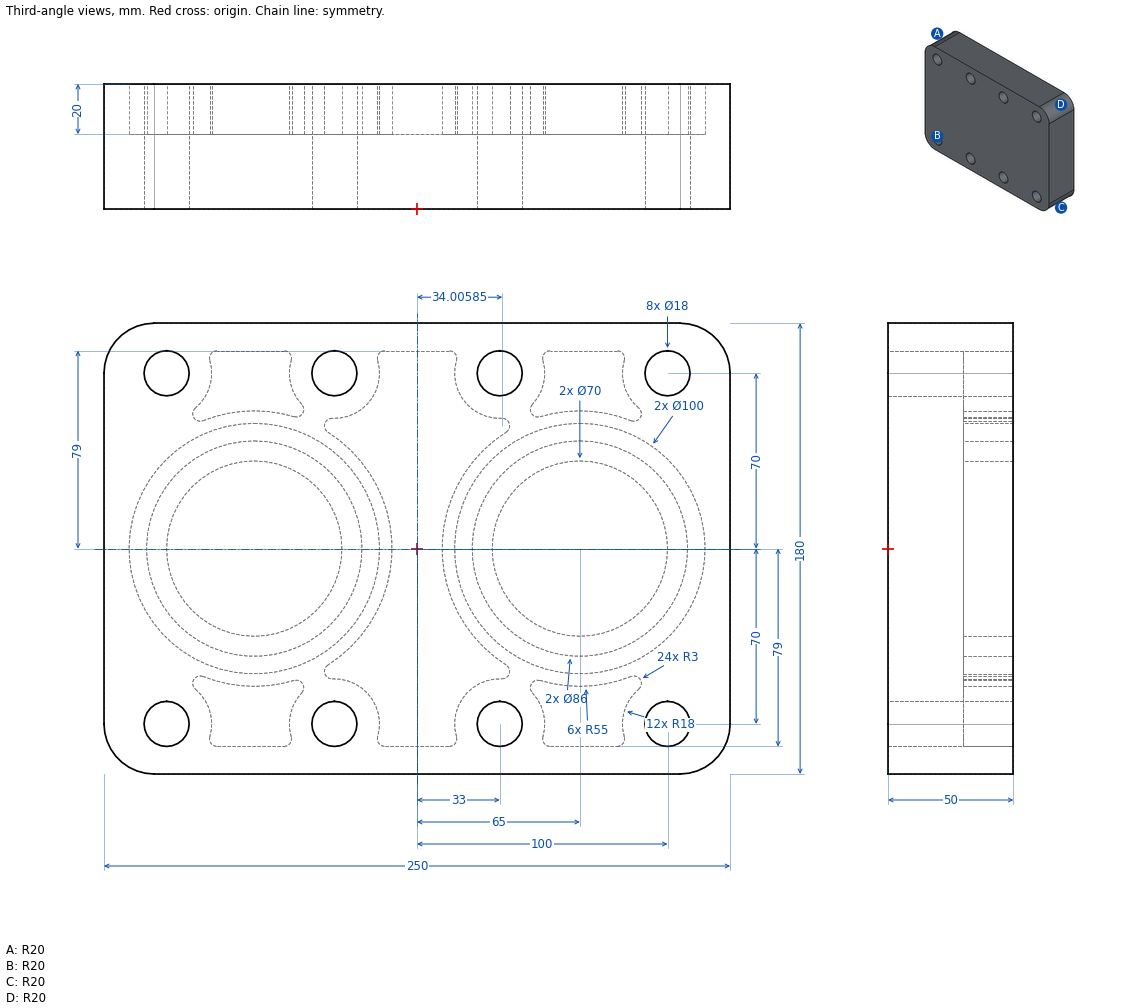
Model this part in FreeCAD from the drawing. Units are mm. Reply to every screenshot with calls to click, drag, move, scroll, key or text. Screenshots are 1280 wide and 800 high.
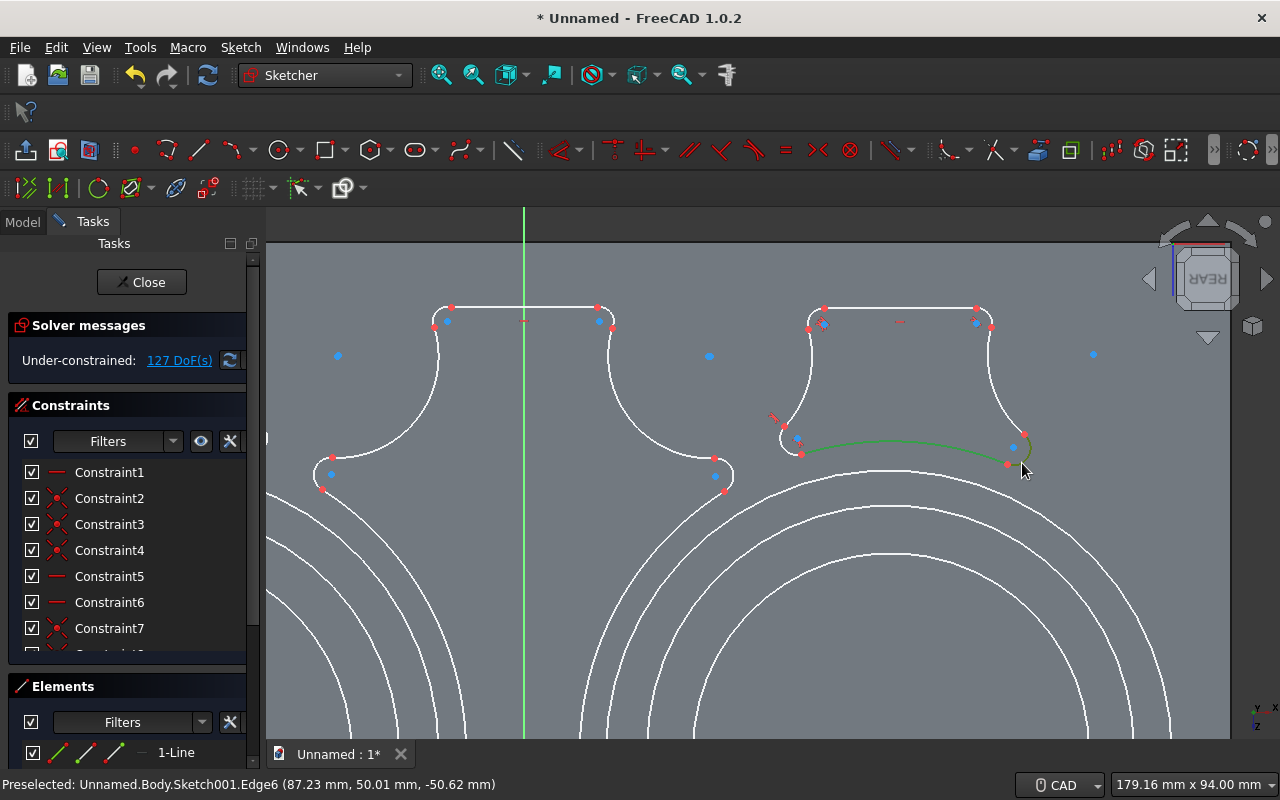
click(754, 150)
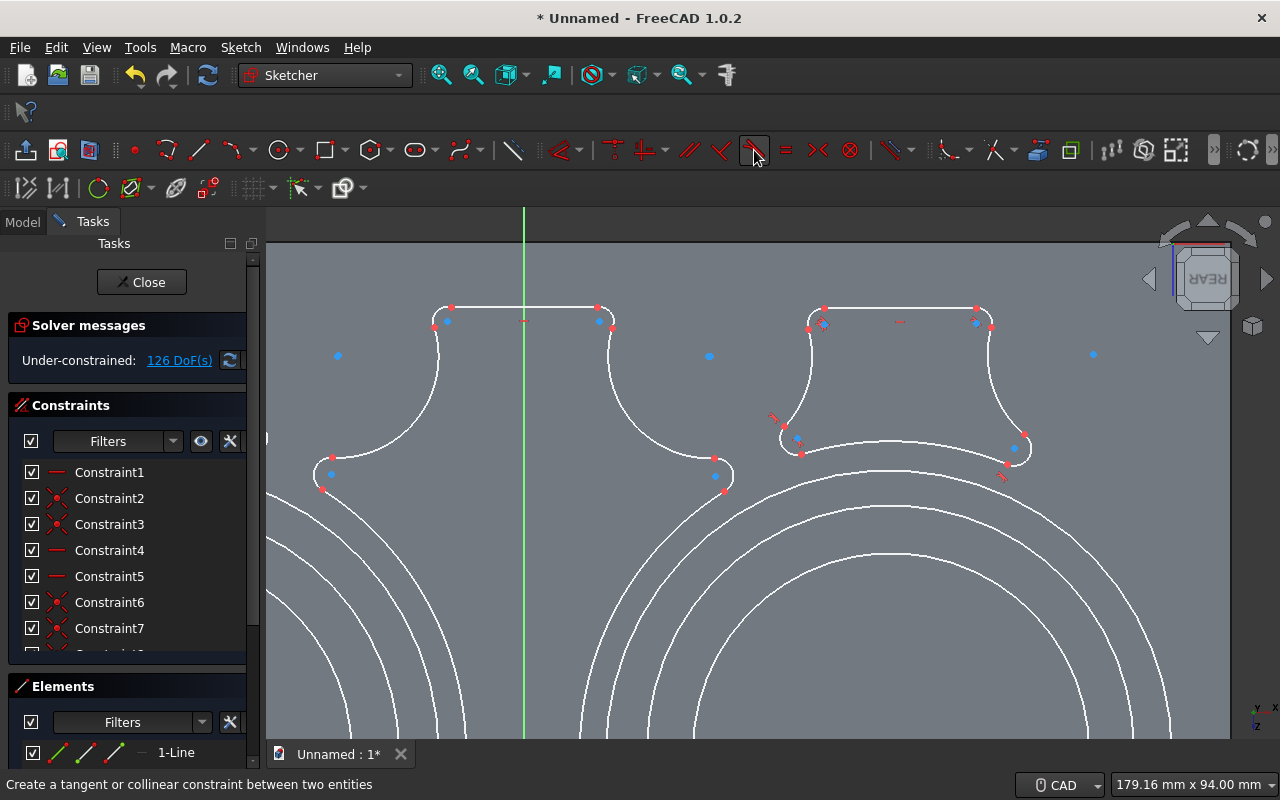
click(1022, 464)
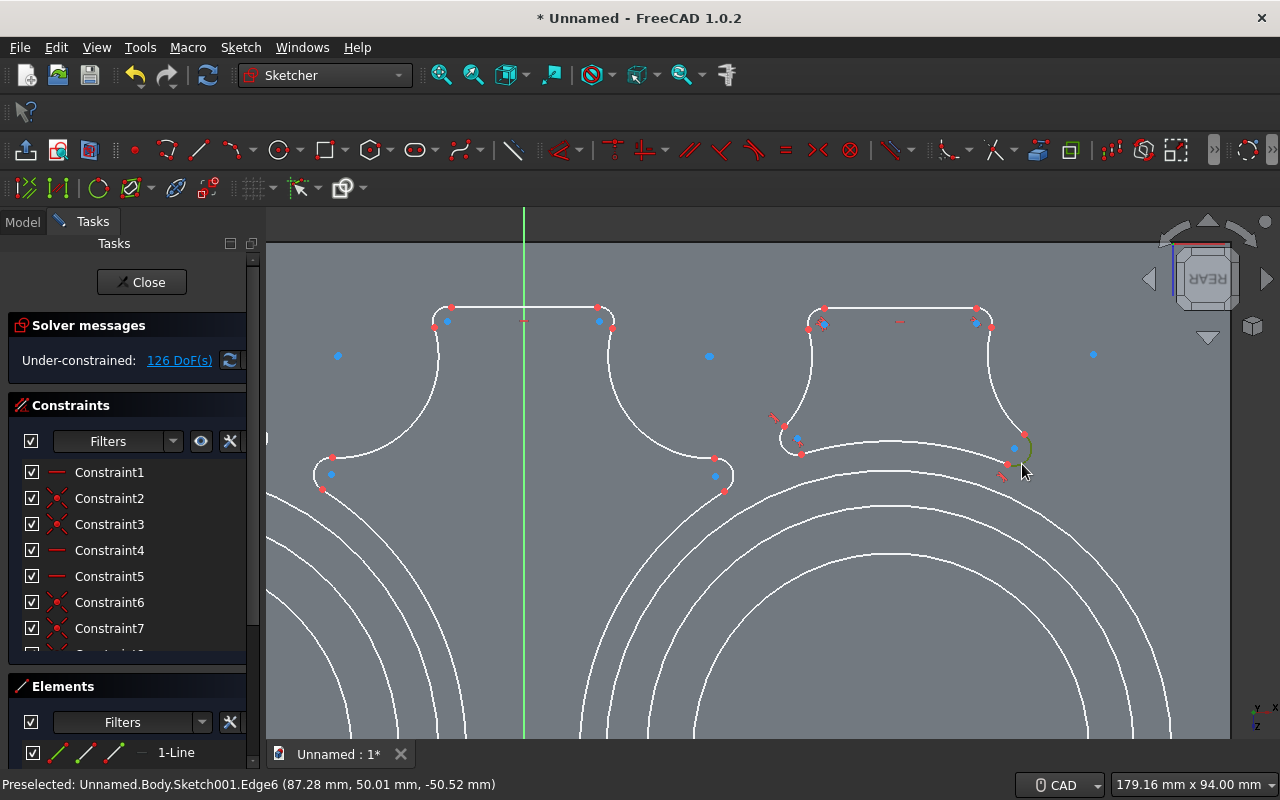
click(988, 362)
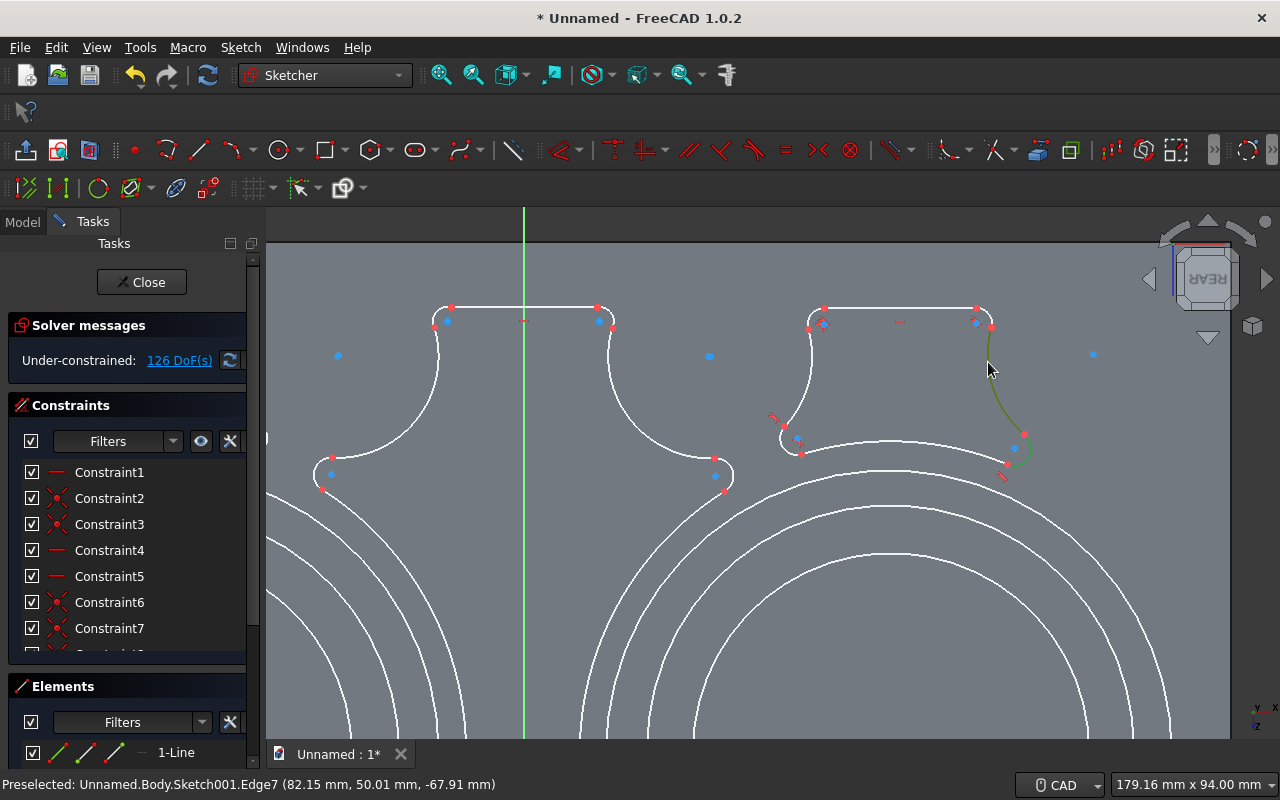
click(754, 150)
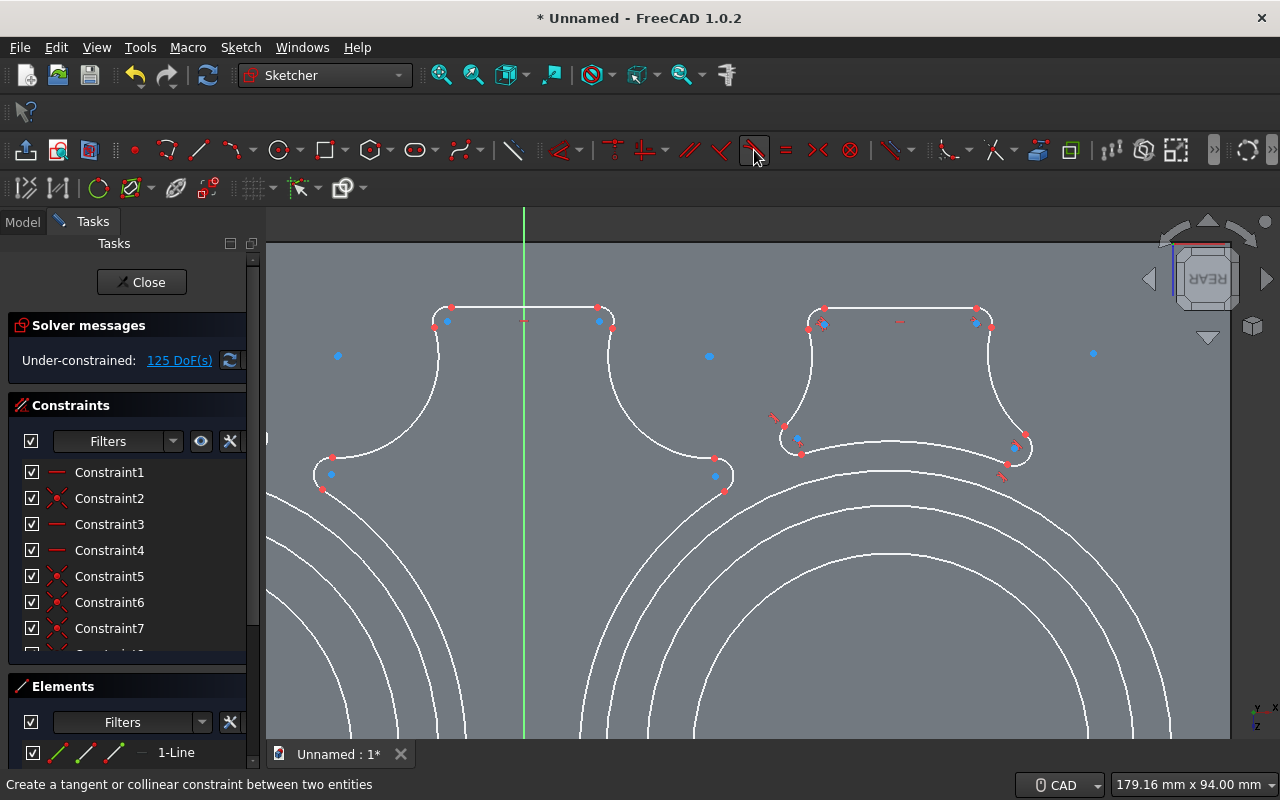
click(988, 362)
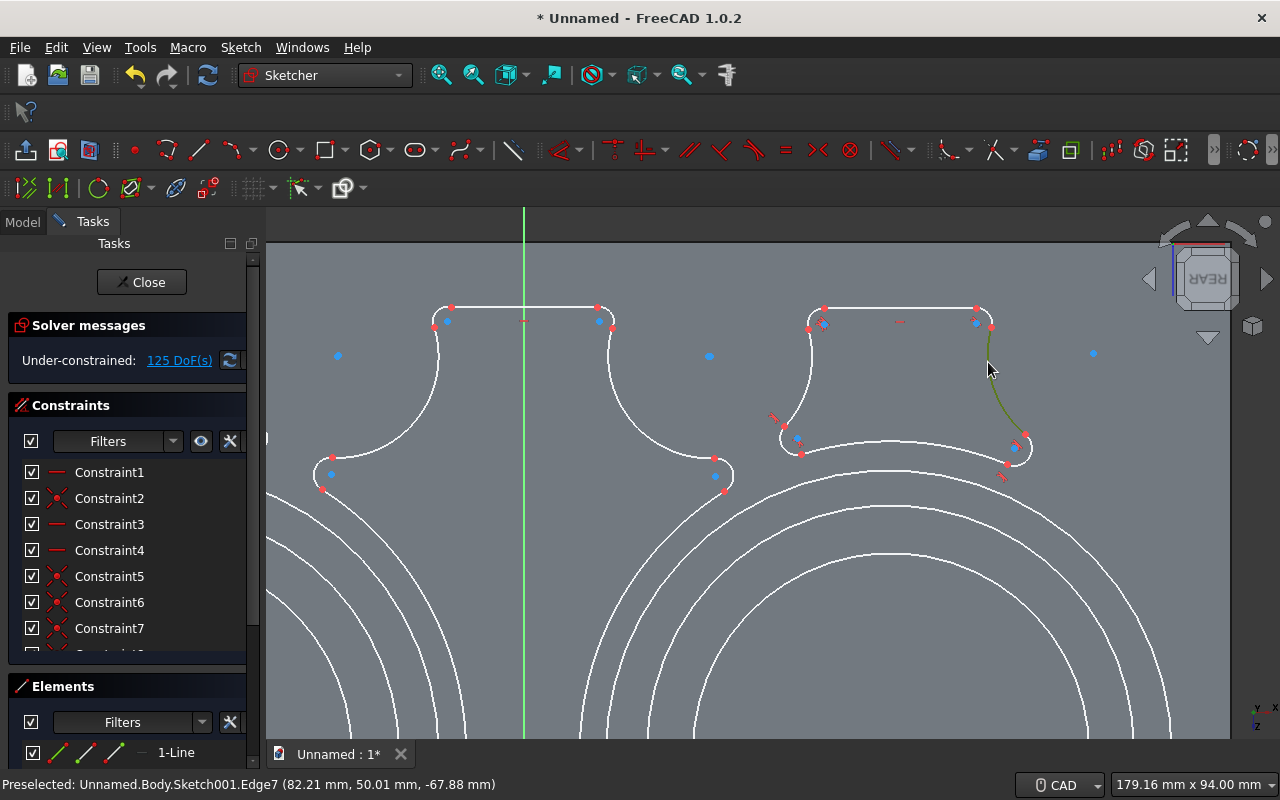
click(989, 314)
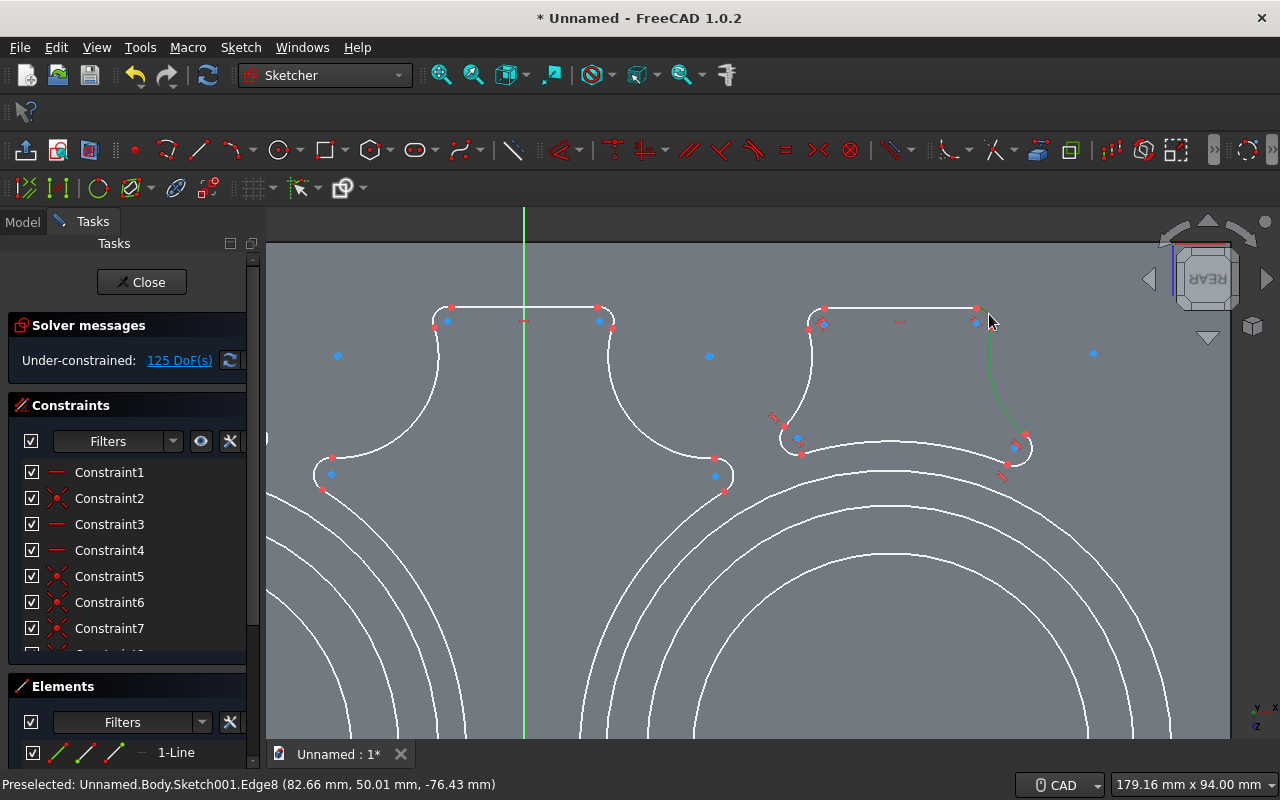
click(754, 150)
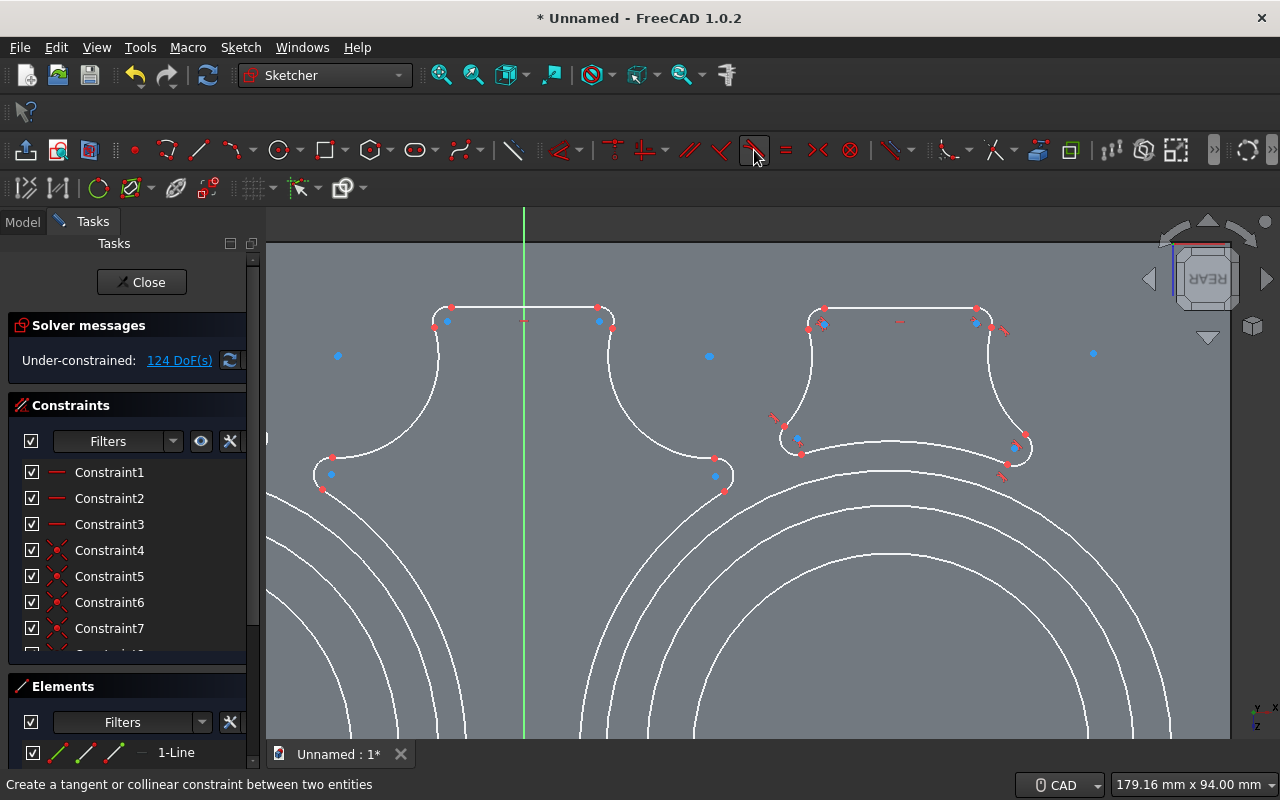
scroll(810, 311, down, 5)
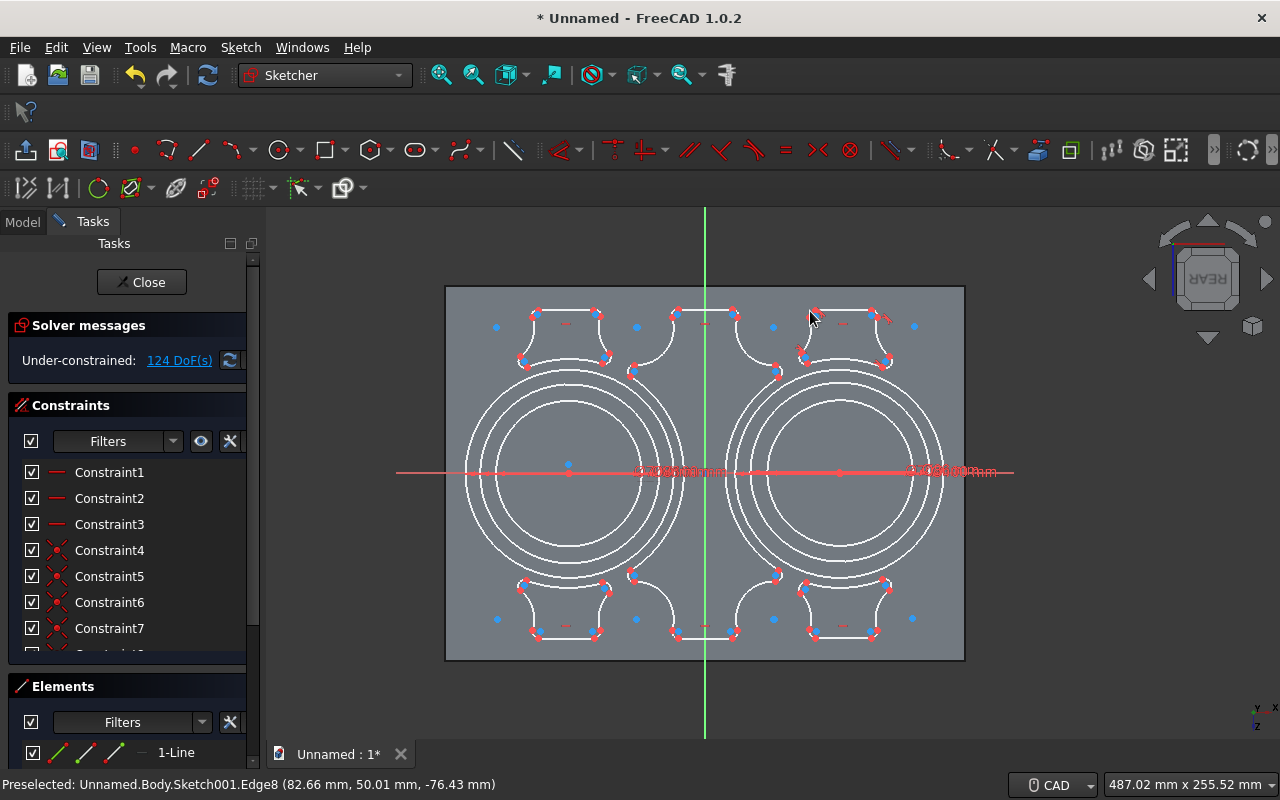
scroll(694, 639, up, 2)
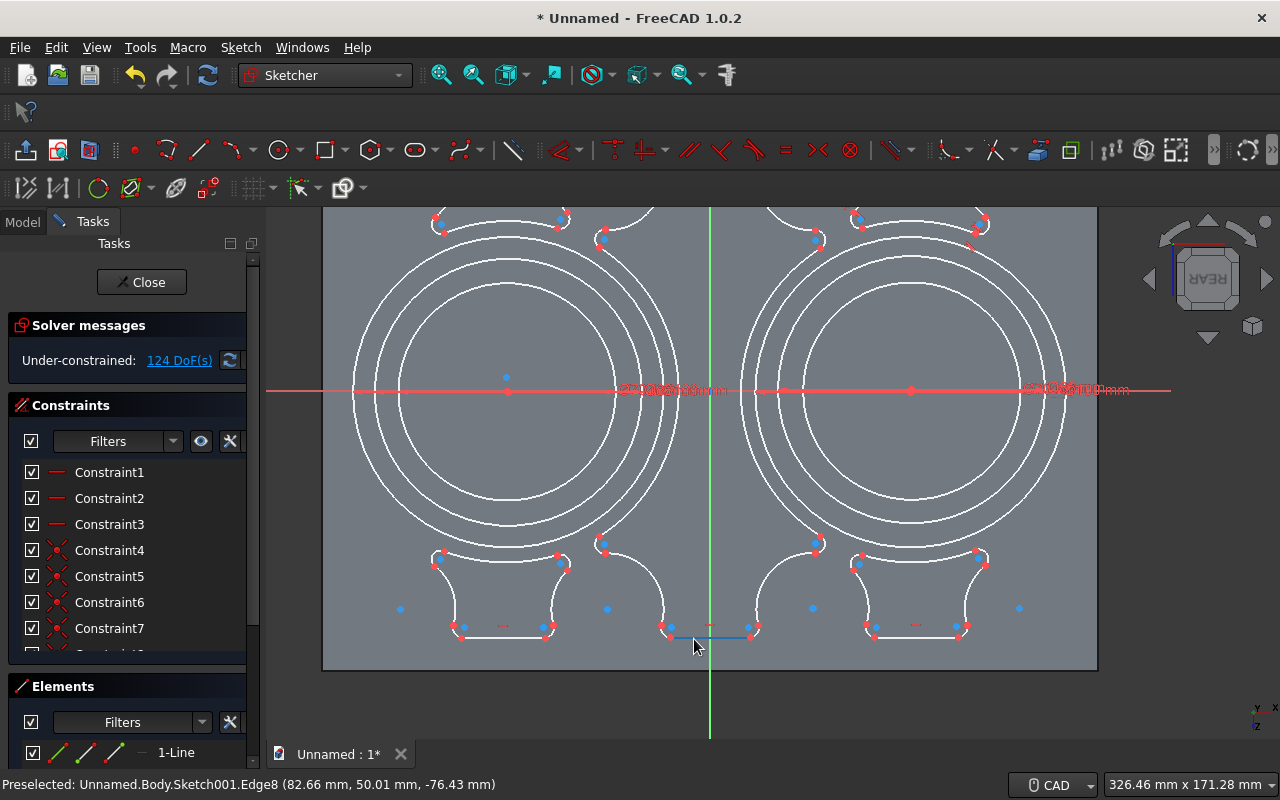
click(694, 638)